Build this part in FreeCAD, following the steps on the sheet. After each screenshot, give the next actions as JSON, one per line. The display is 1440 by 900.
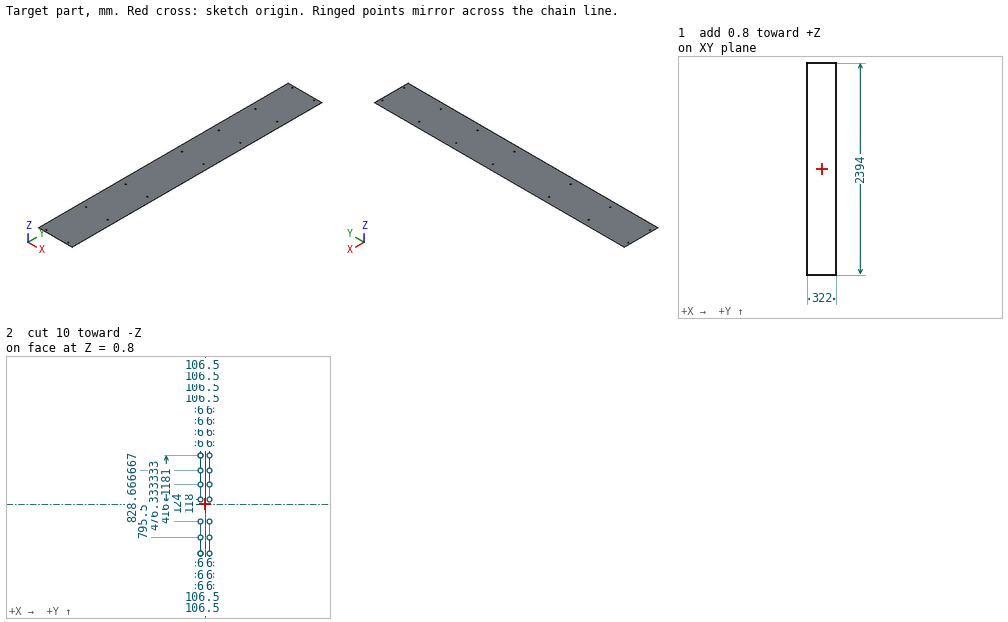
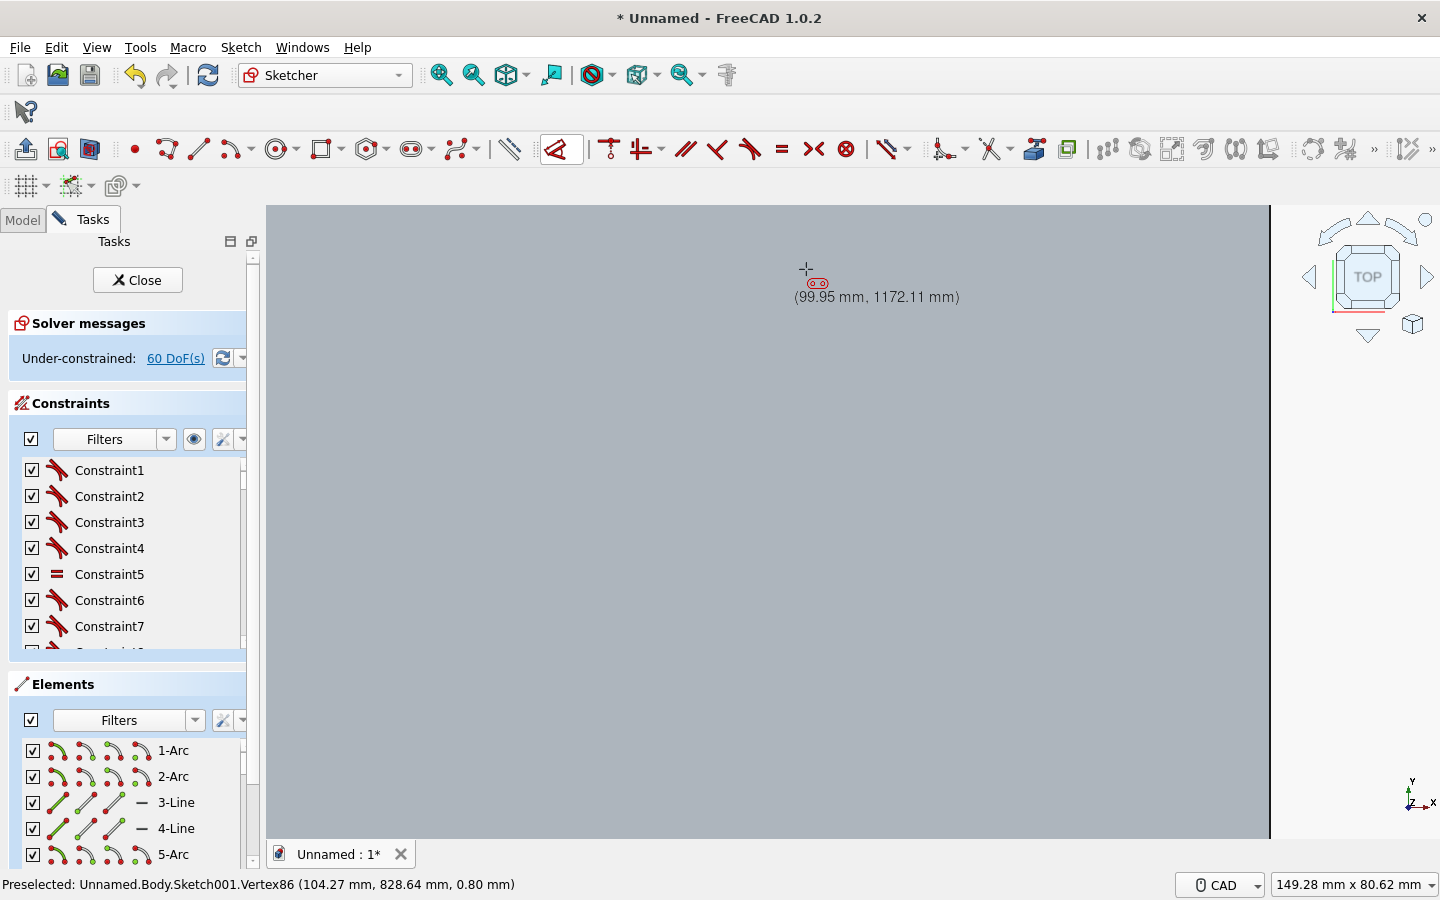
{"action": "scroll", "coordinate": [806, 269], "scroll_direction": "down", "scroll_amount": 18}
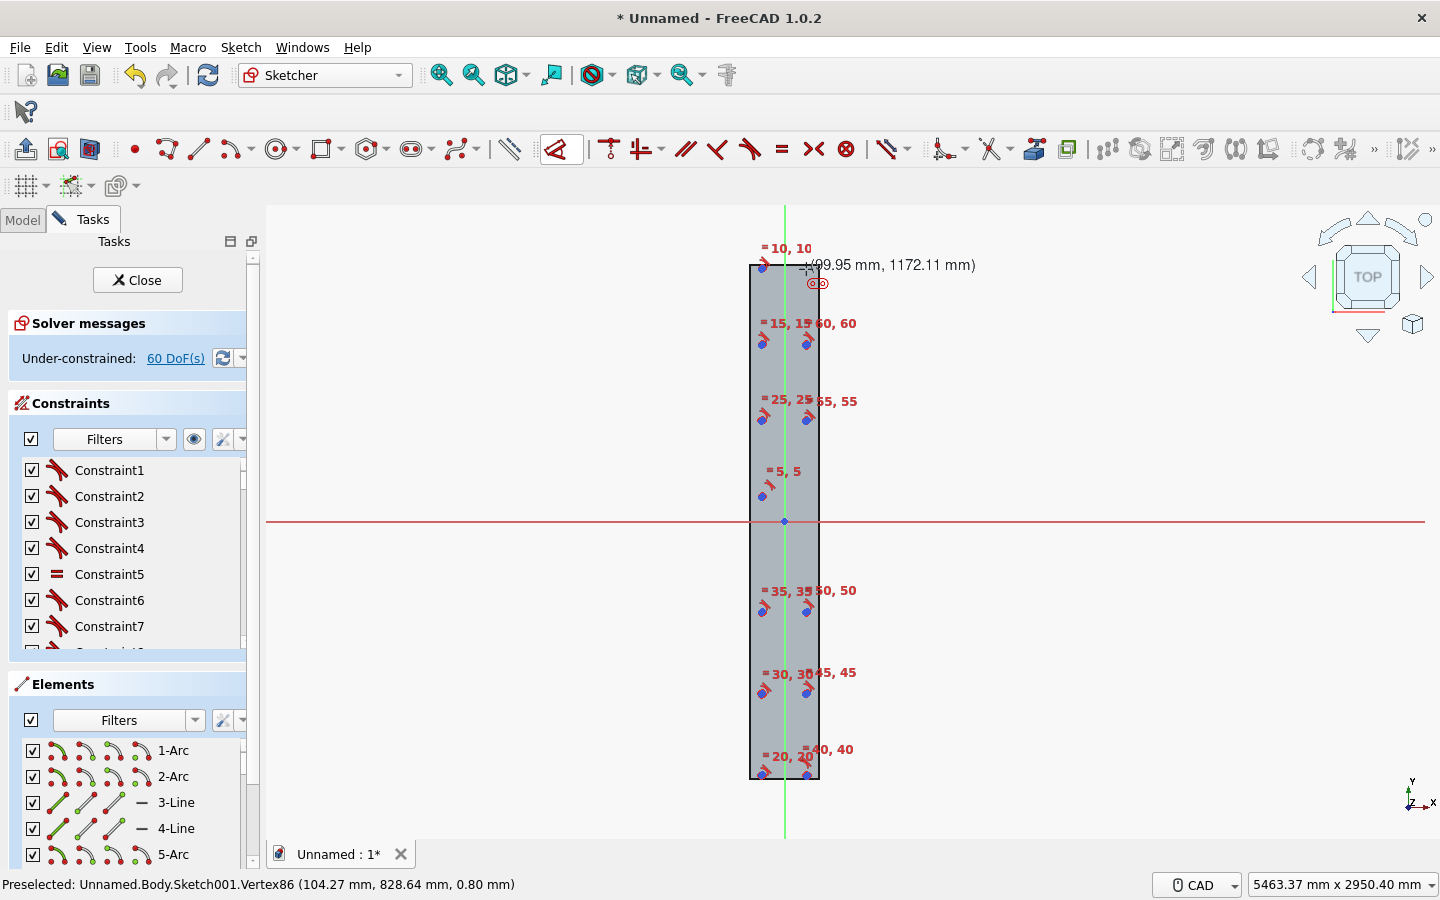
{"action": "left_click", "coordinate": [806, 269]}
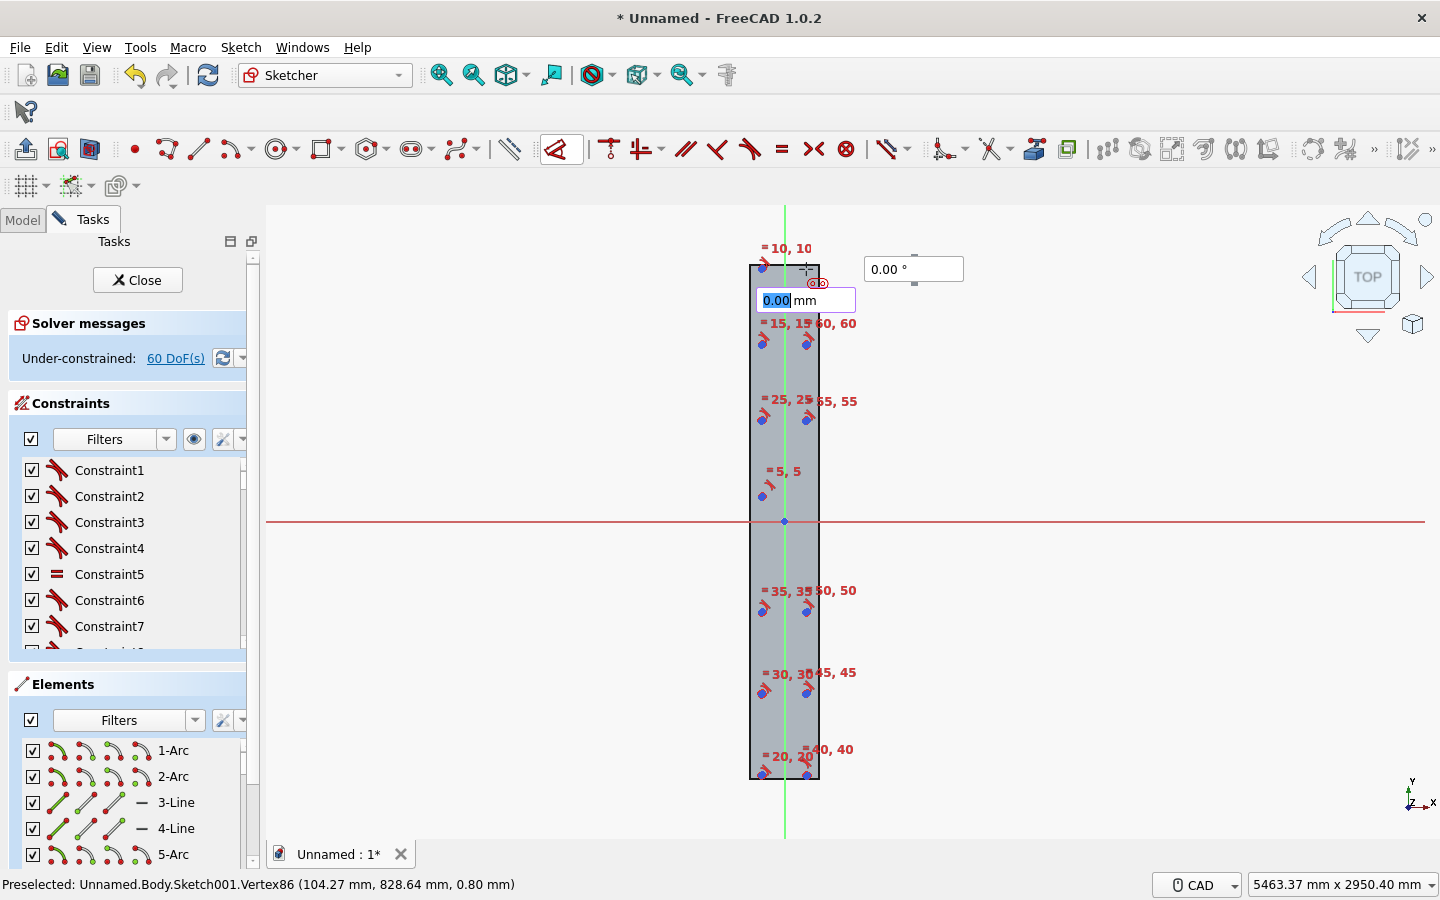
{"action": "scroll", "coordinate": [807, 269], "scroll_direction": "up", "scroll_amount": 13}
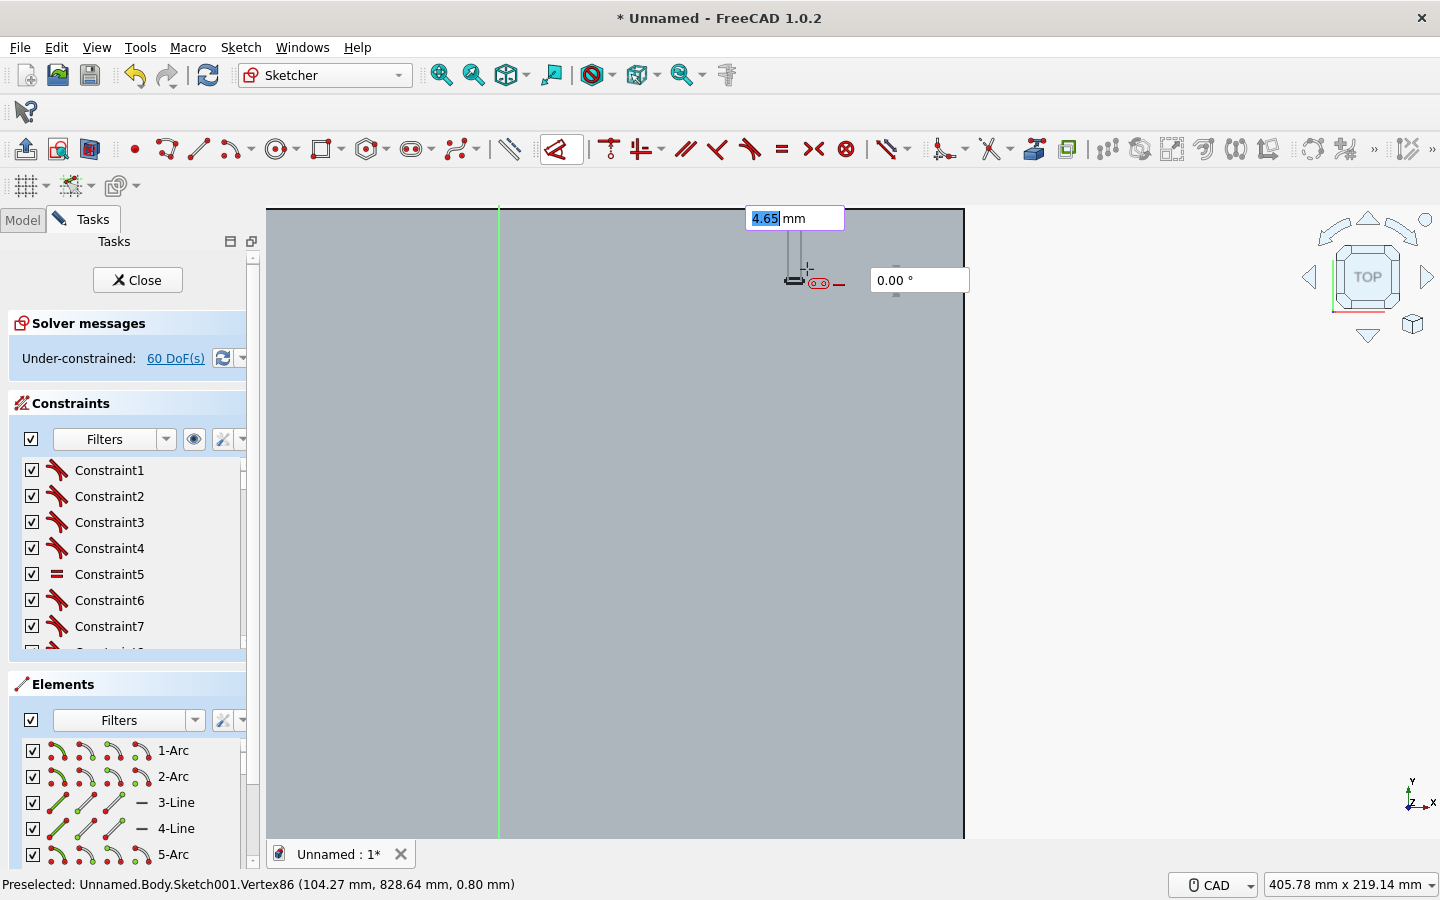
{"action": "left_click", "coordinate": [807, 268]}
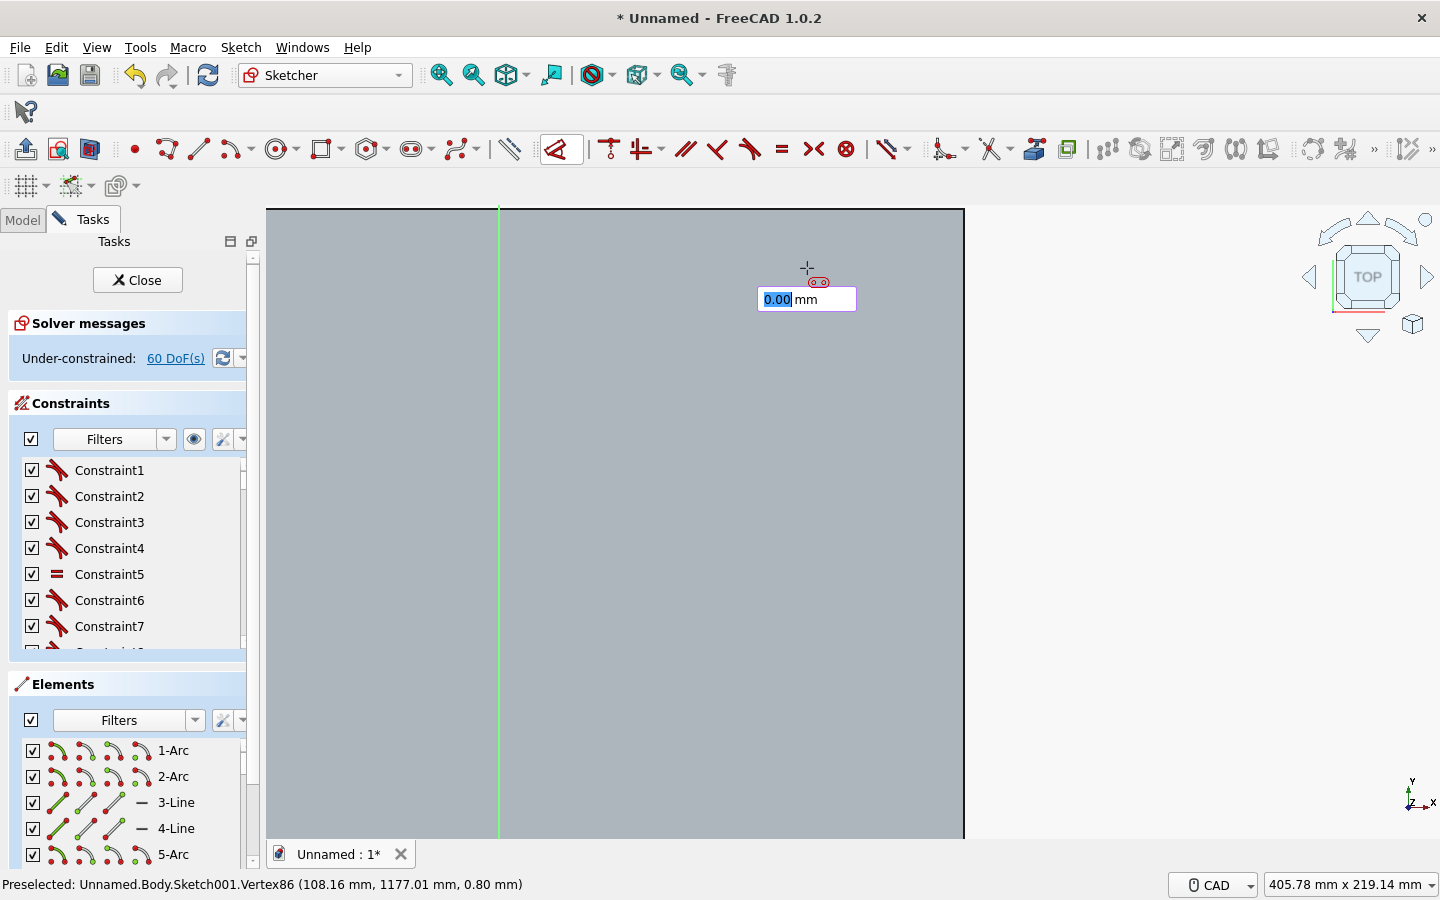
{"action": "scroll", "coordinate": [798, 255], "scroll_direction": "up", "scroll_amount": 4}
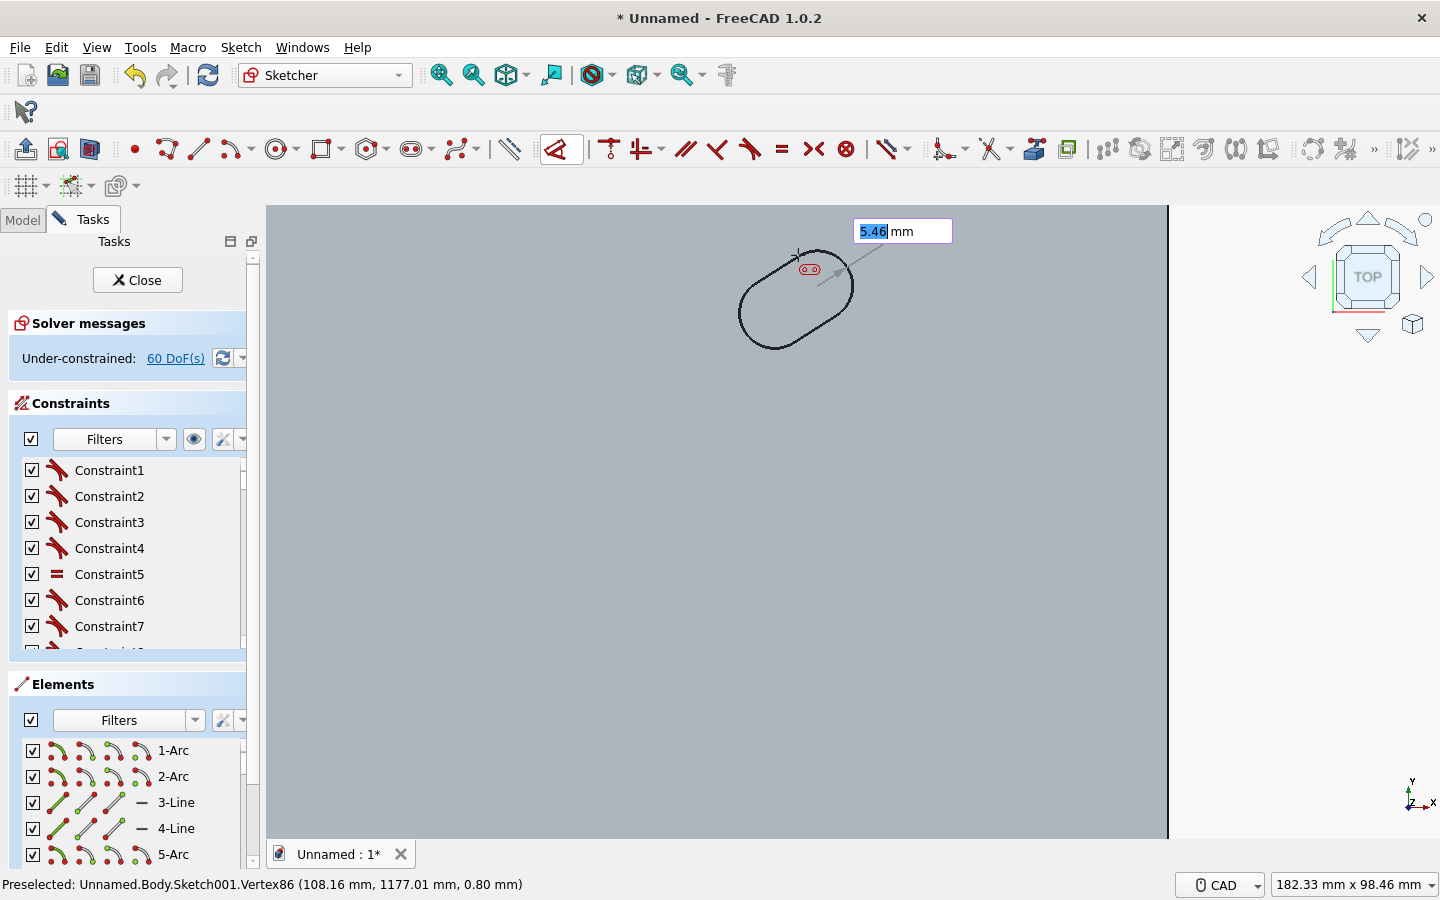
{"action": "left_click", "coordinate": [798, 256]}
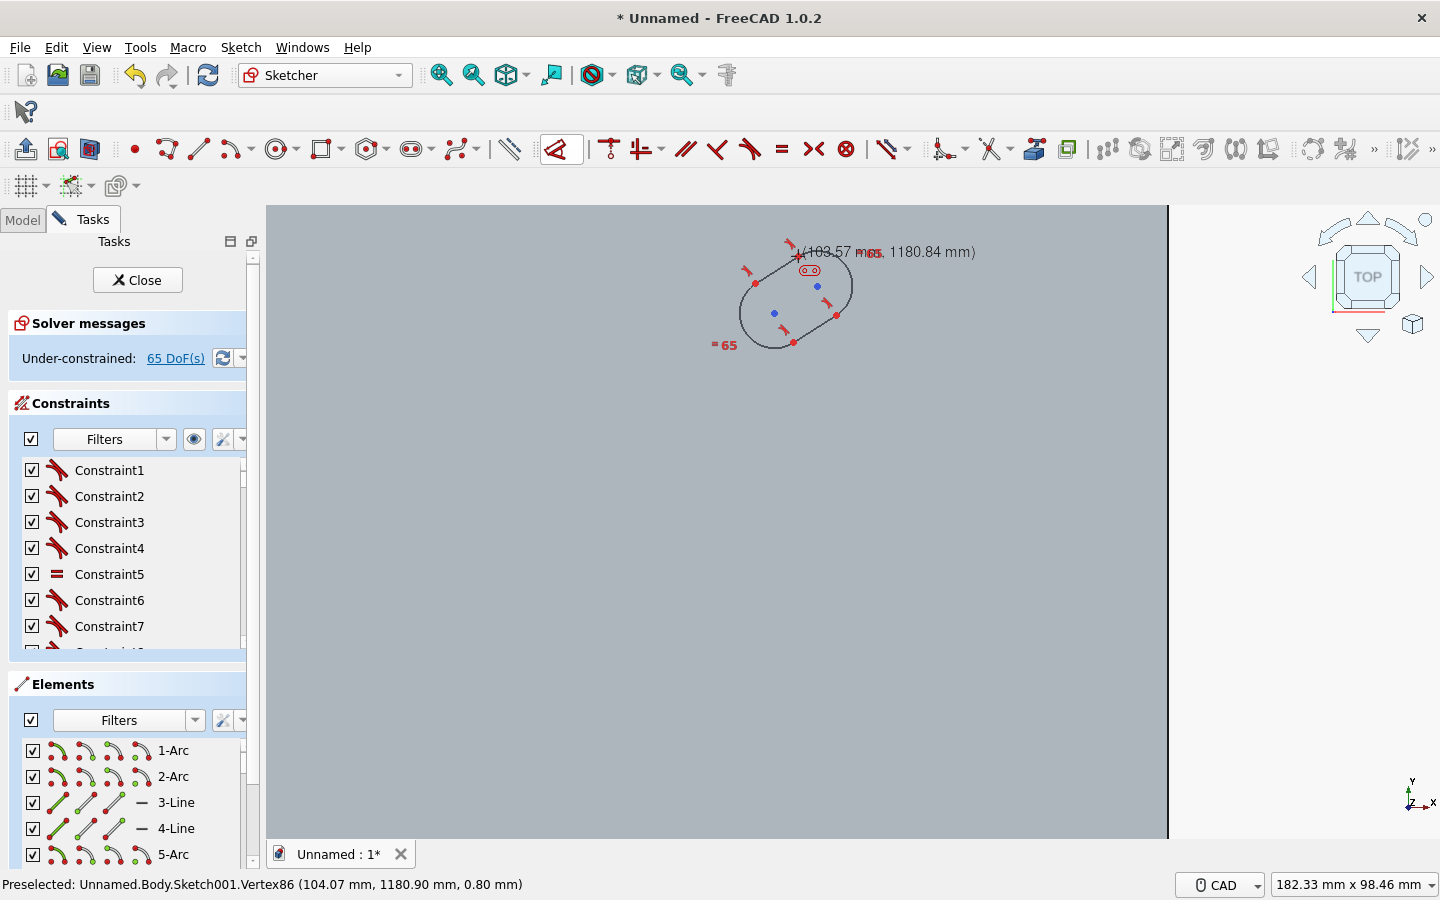
{"action": "scroll", "coordinate": [807, 269], "scroll_direction": "down", "scroll_amount": 17}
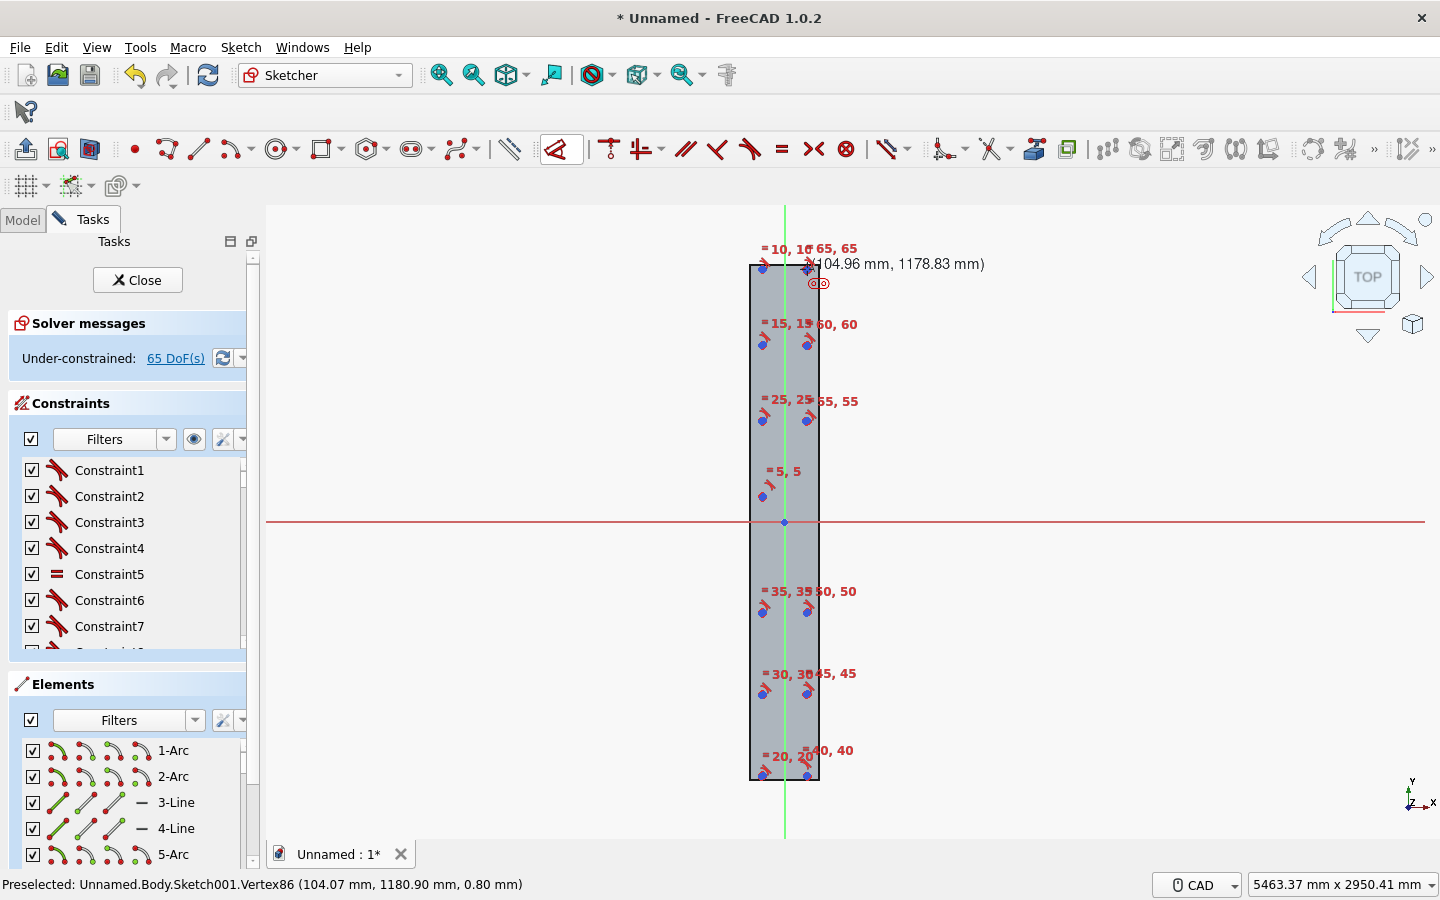
{"action": "scroll", "coordinate": [806, 496], "scroll_direction": "up", "scroll_amount": 18}